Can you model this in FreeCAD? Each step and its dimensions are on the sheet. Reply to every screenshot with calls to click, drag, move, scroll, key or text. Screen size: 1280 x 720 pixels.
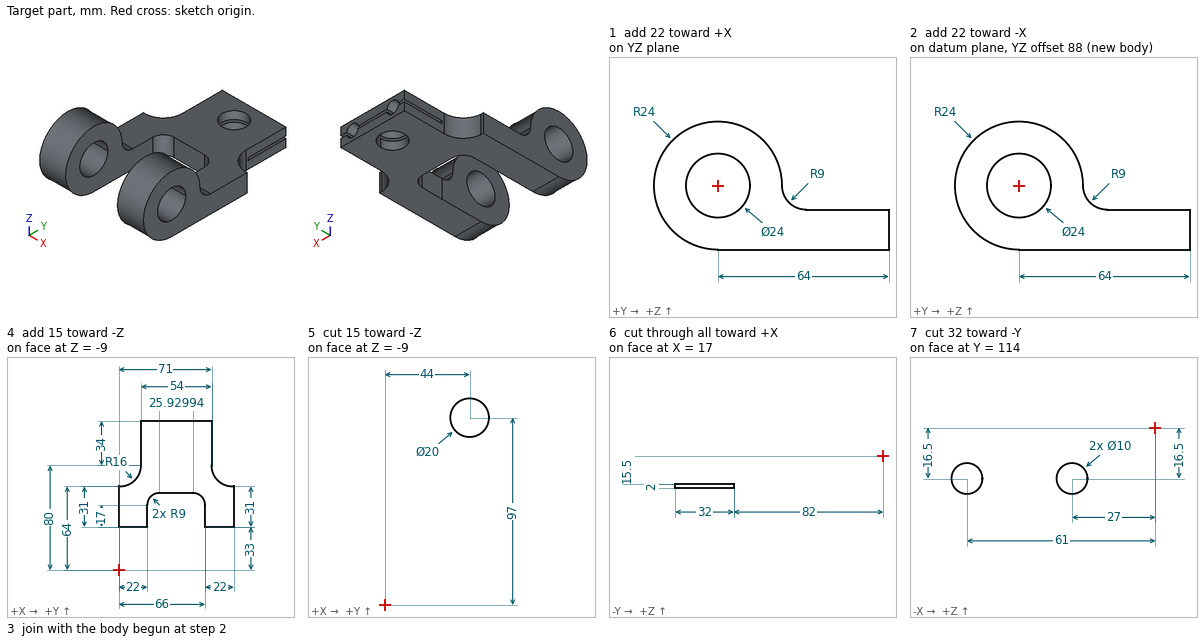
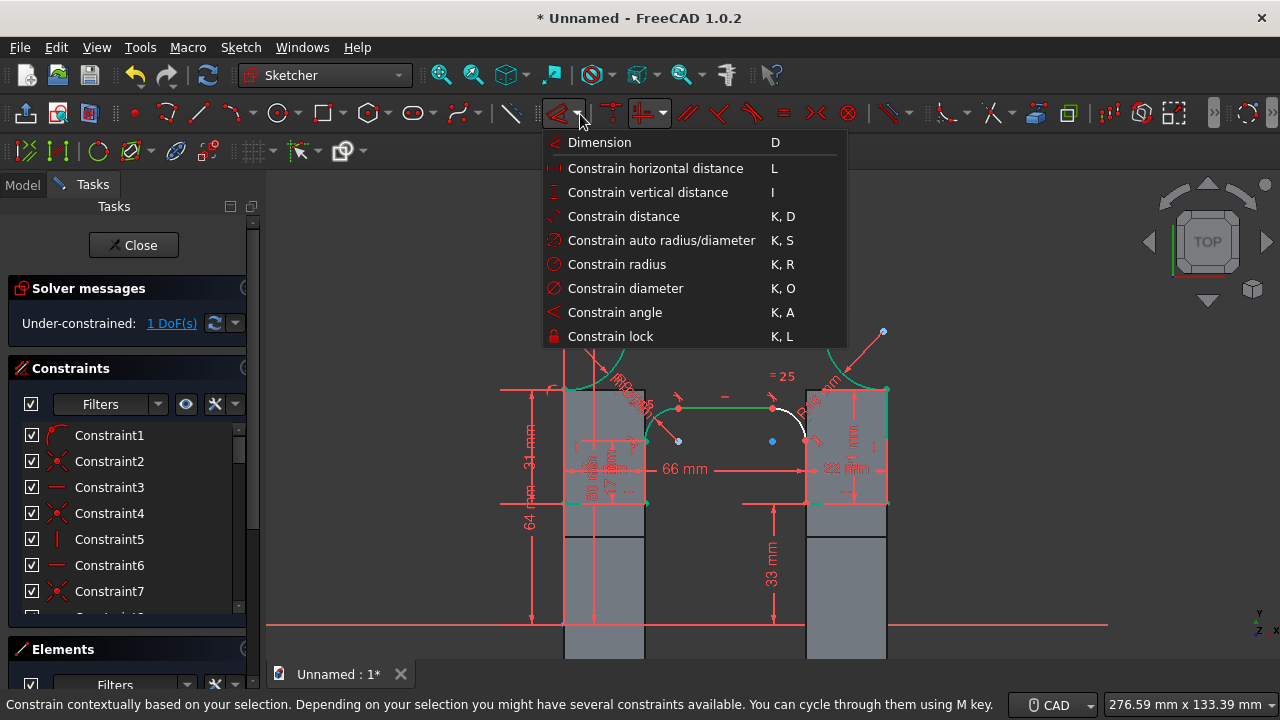
click(695, 168)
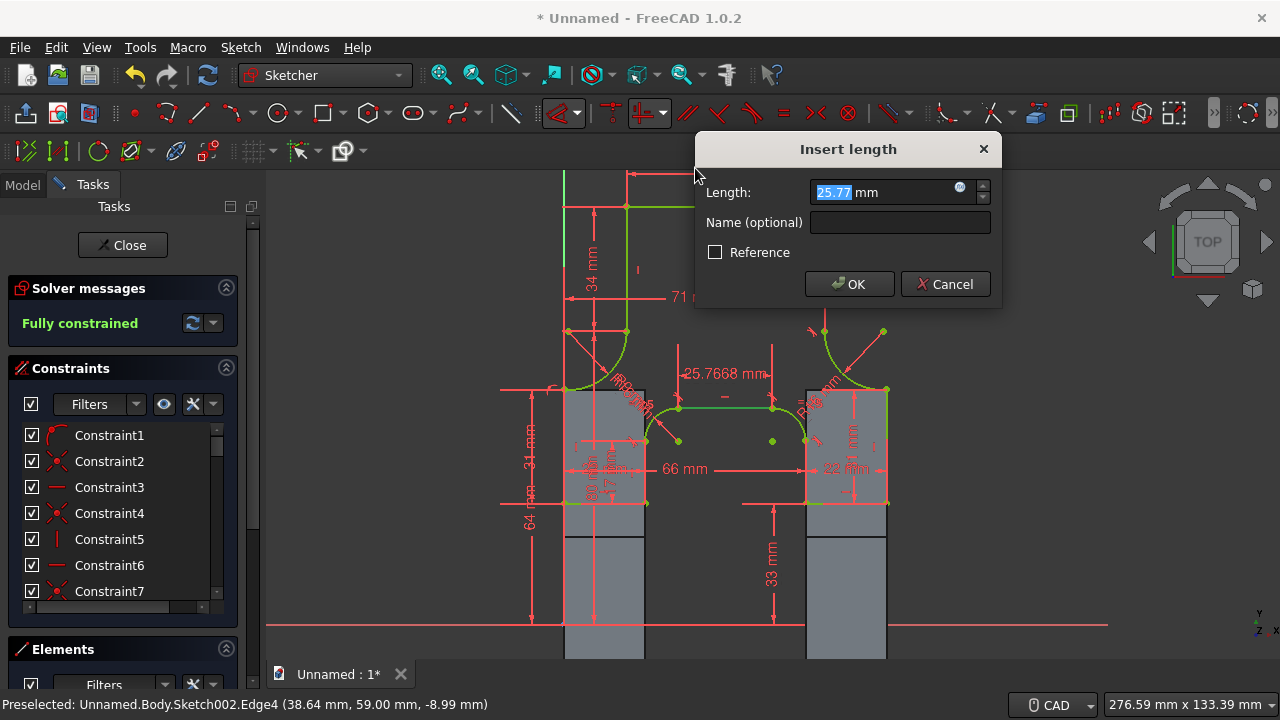
text(25.92994)
key(Return)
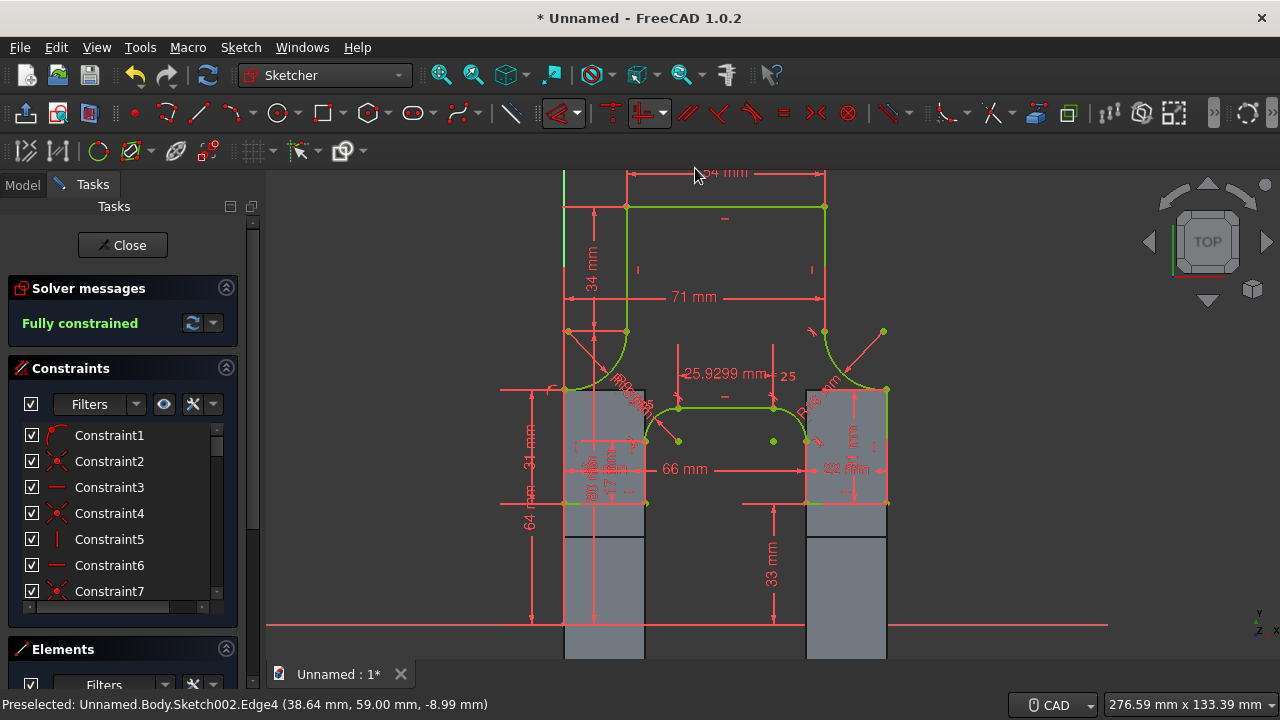
click(123, 245)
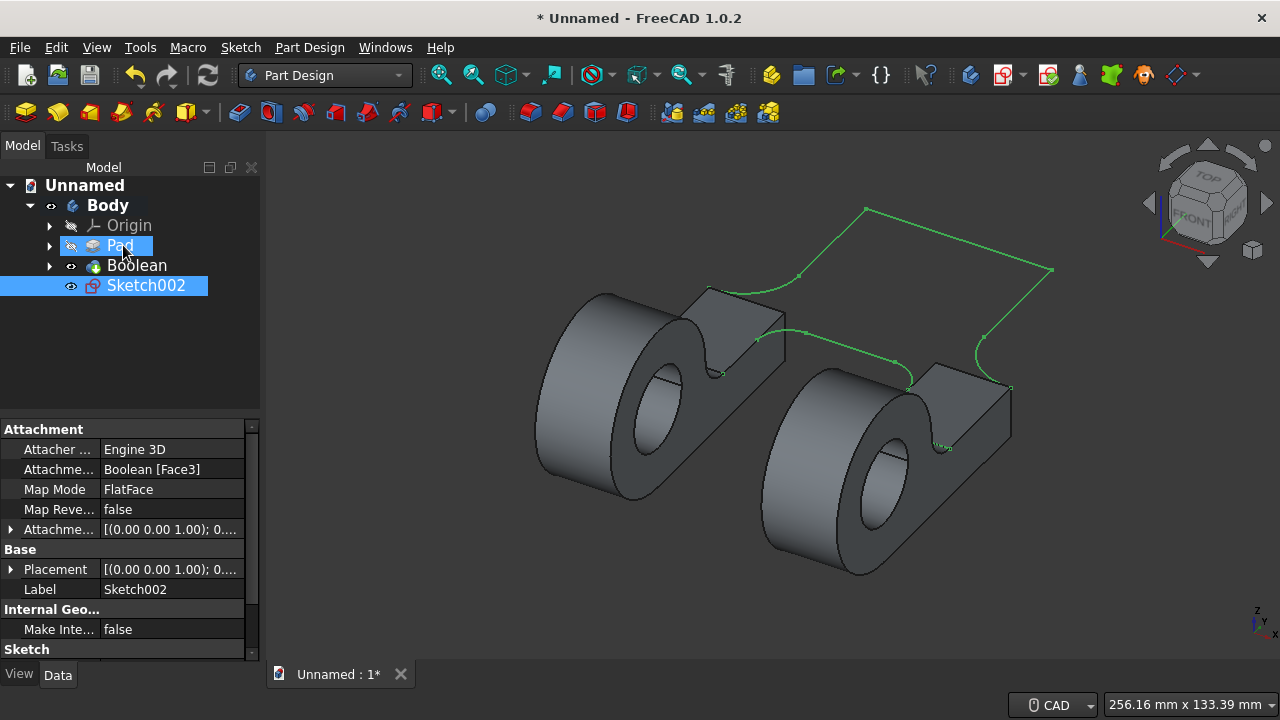
click(26, 112)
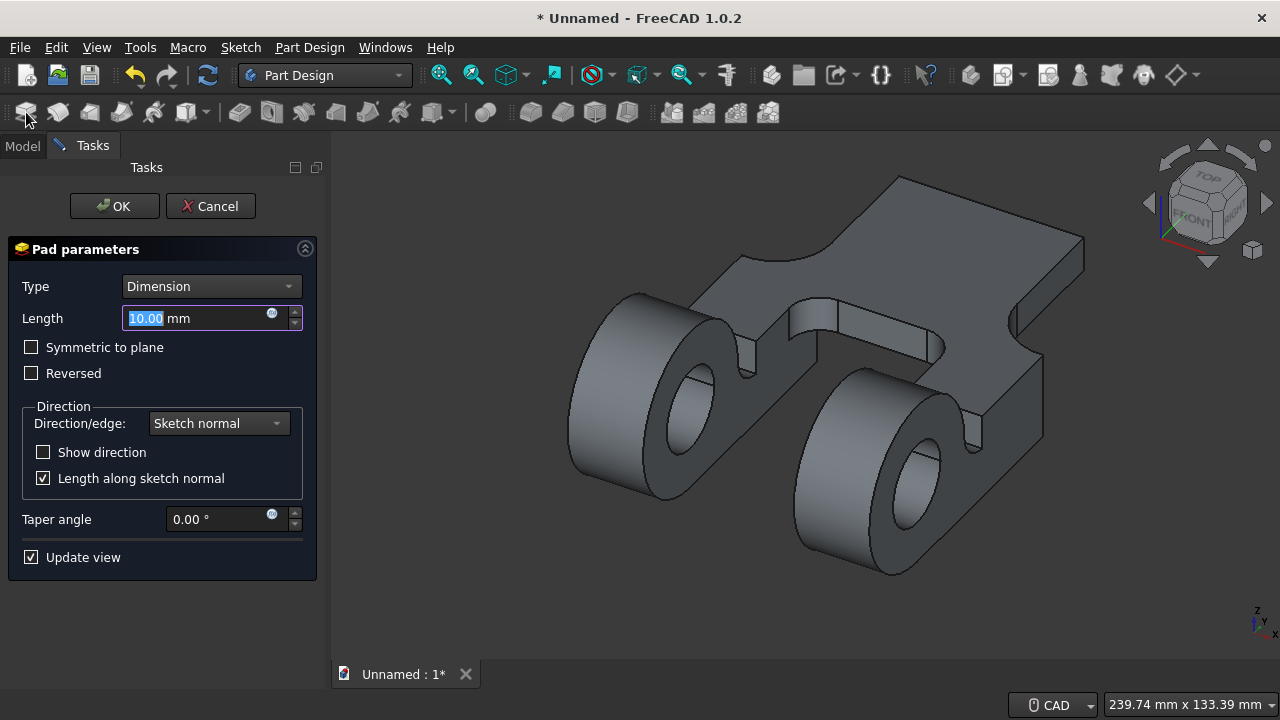
text(15)
key(Tab)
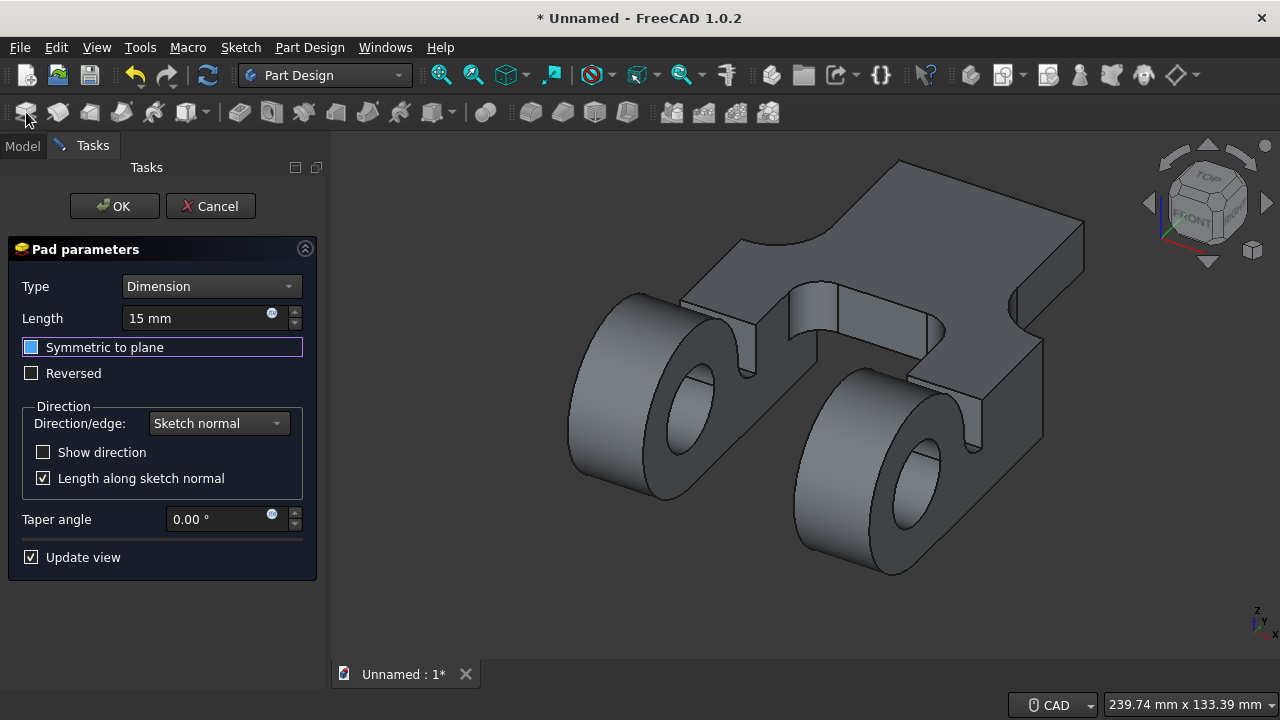
click(30, 373)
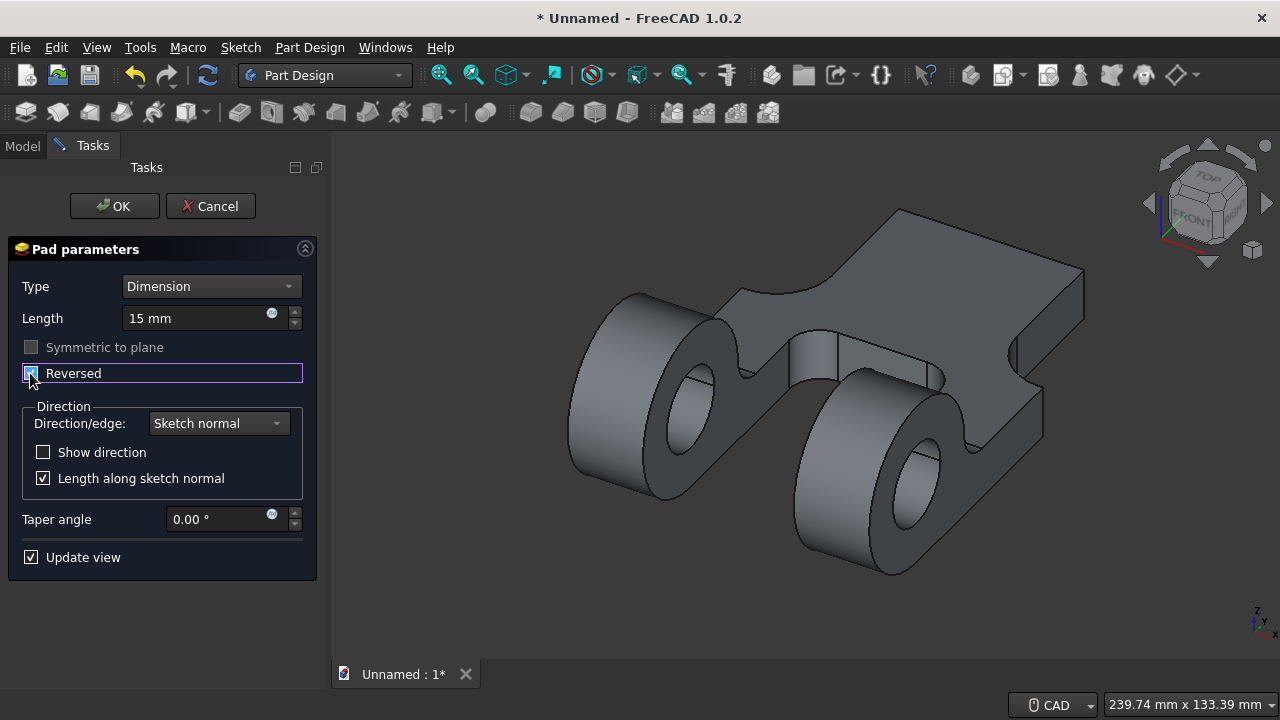
click(115, 206)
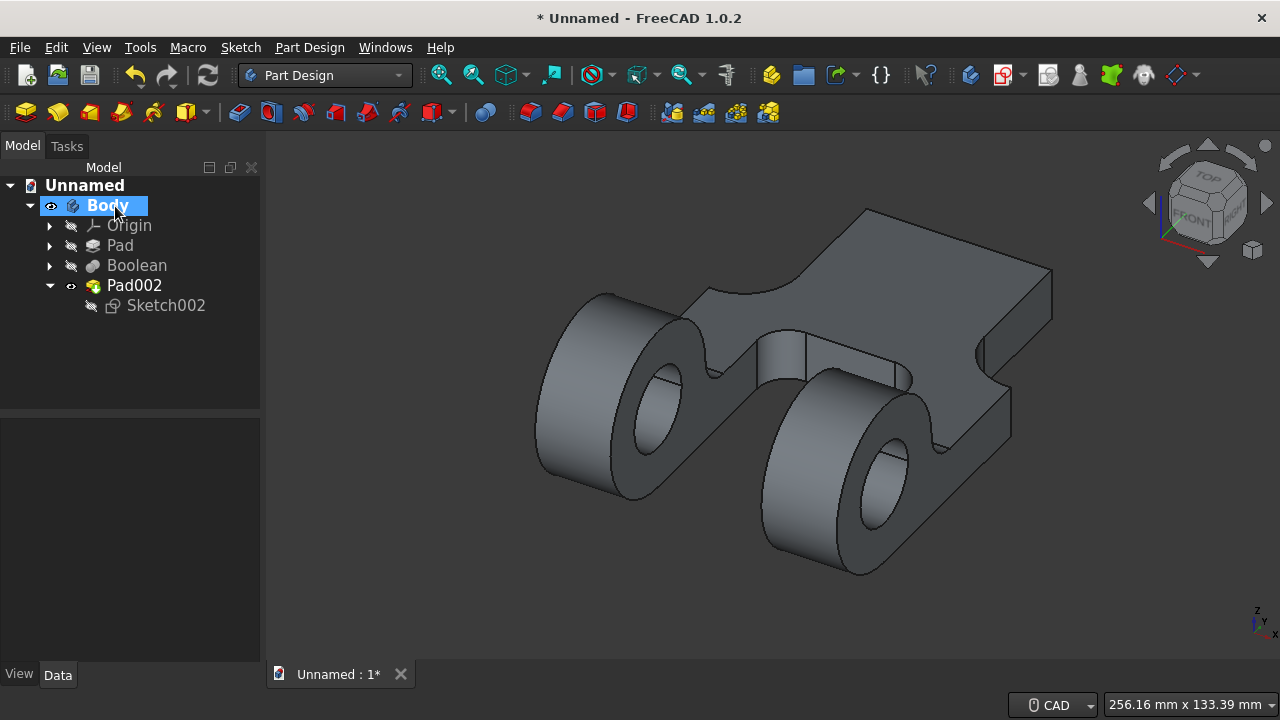
click(442, 76)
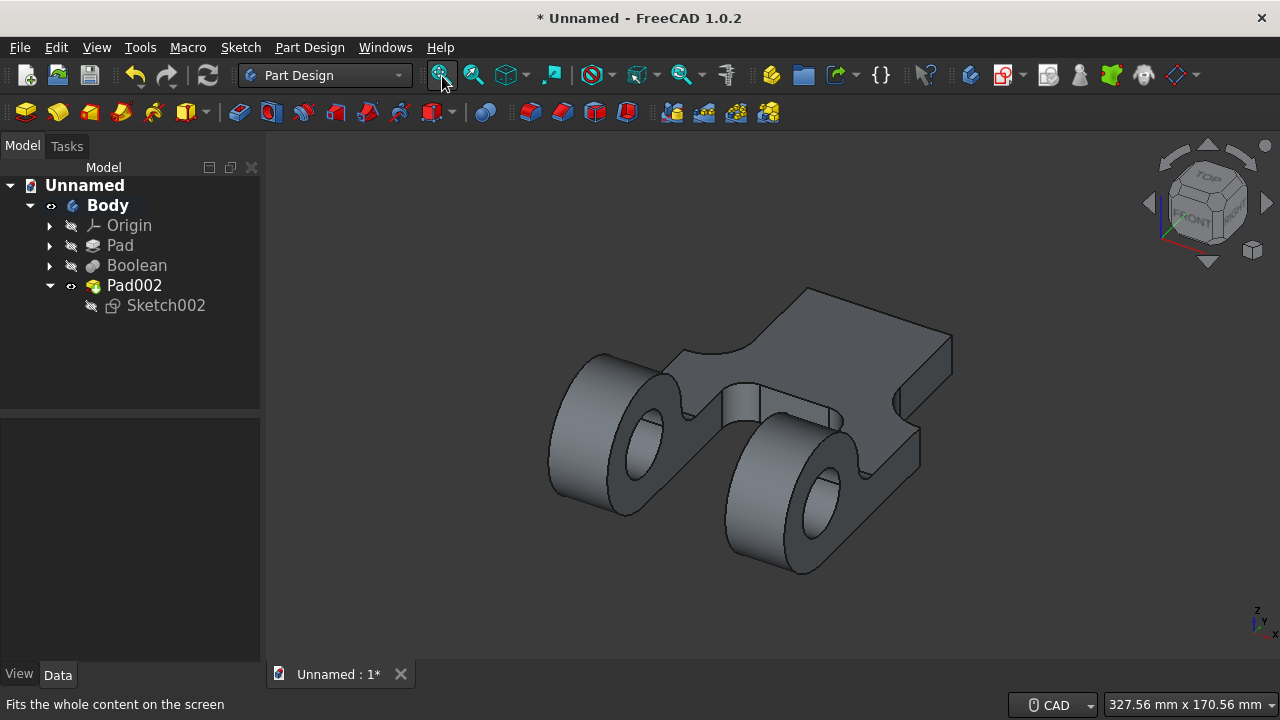
click(835, 355)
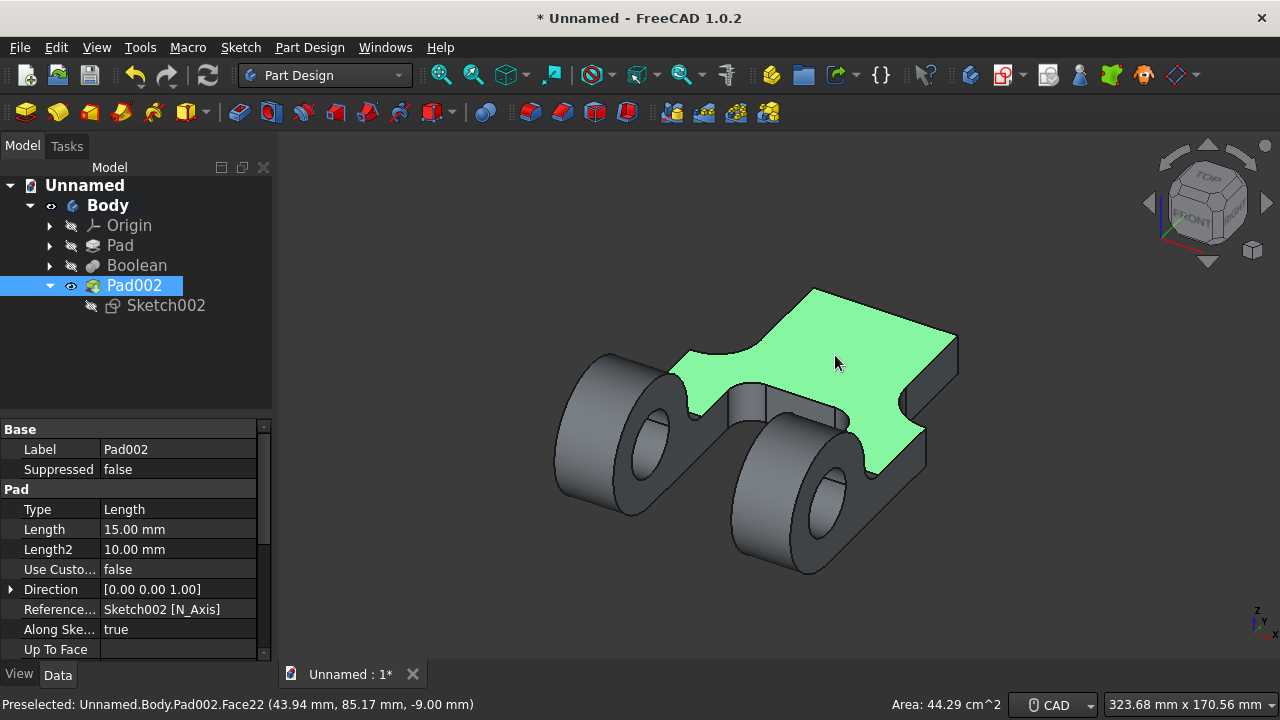
click(1004, 76)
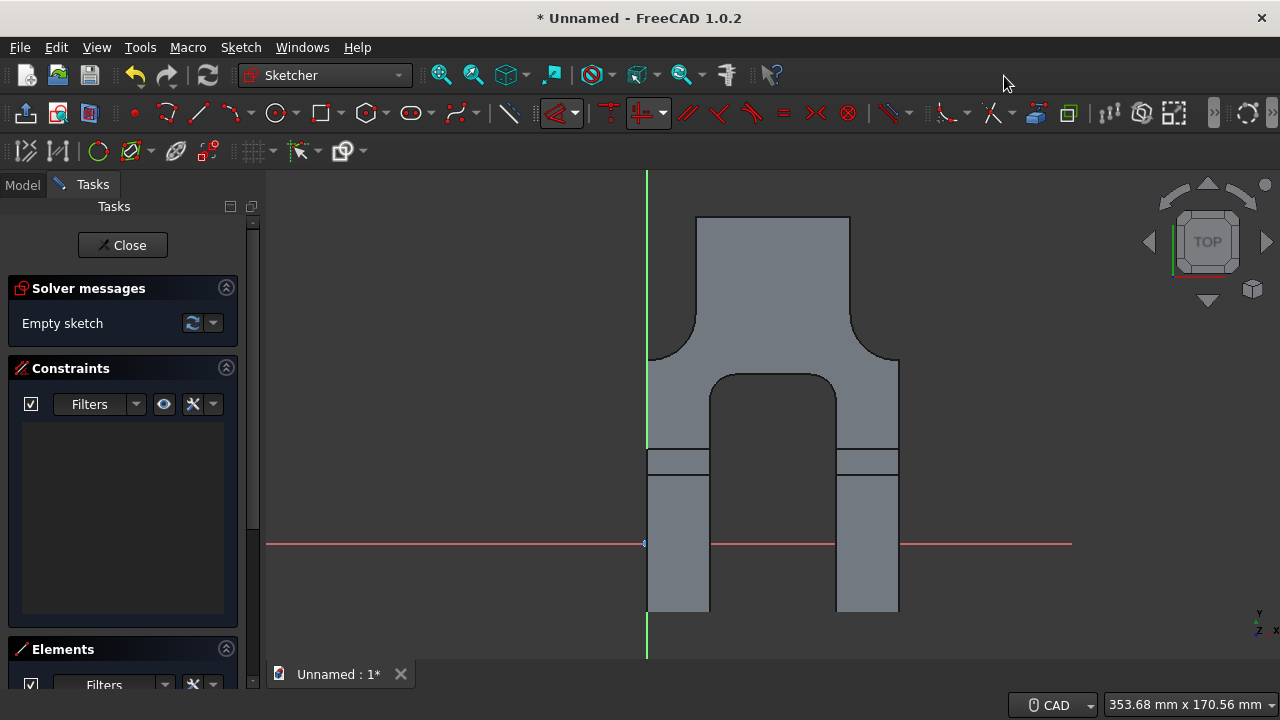
click(90, 114)